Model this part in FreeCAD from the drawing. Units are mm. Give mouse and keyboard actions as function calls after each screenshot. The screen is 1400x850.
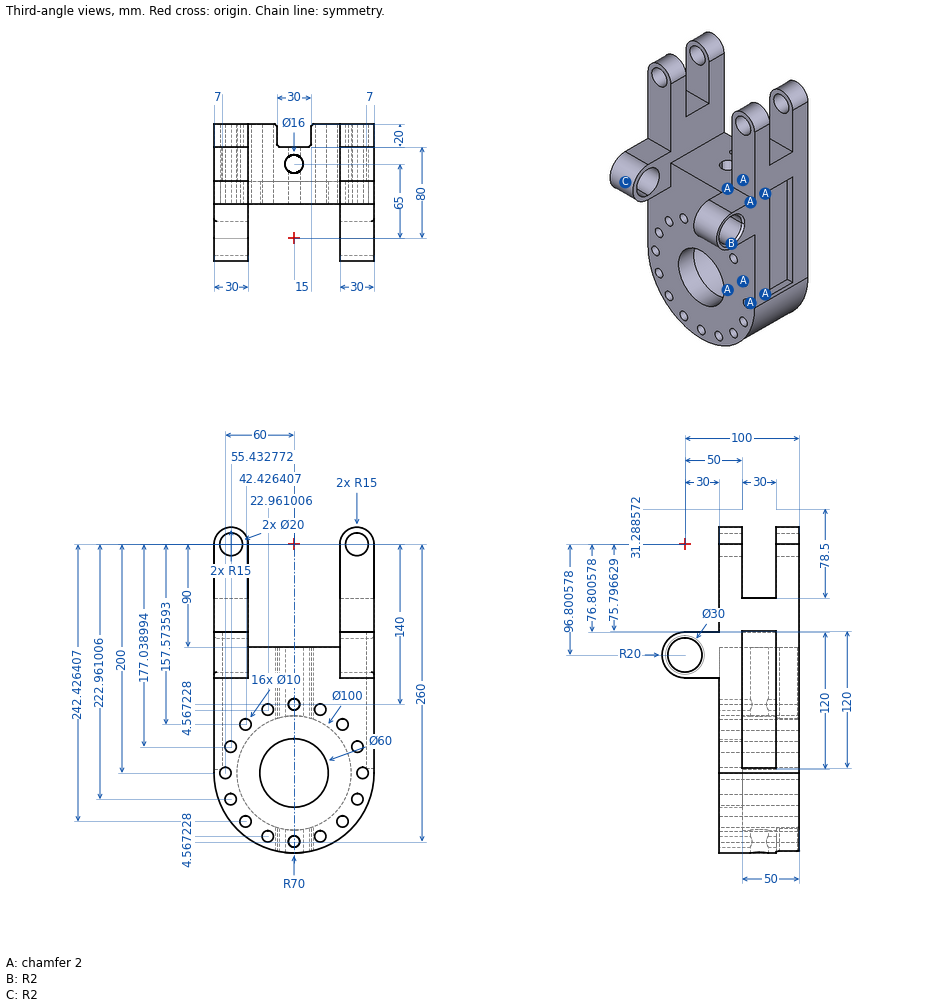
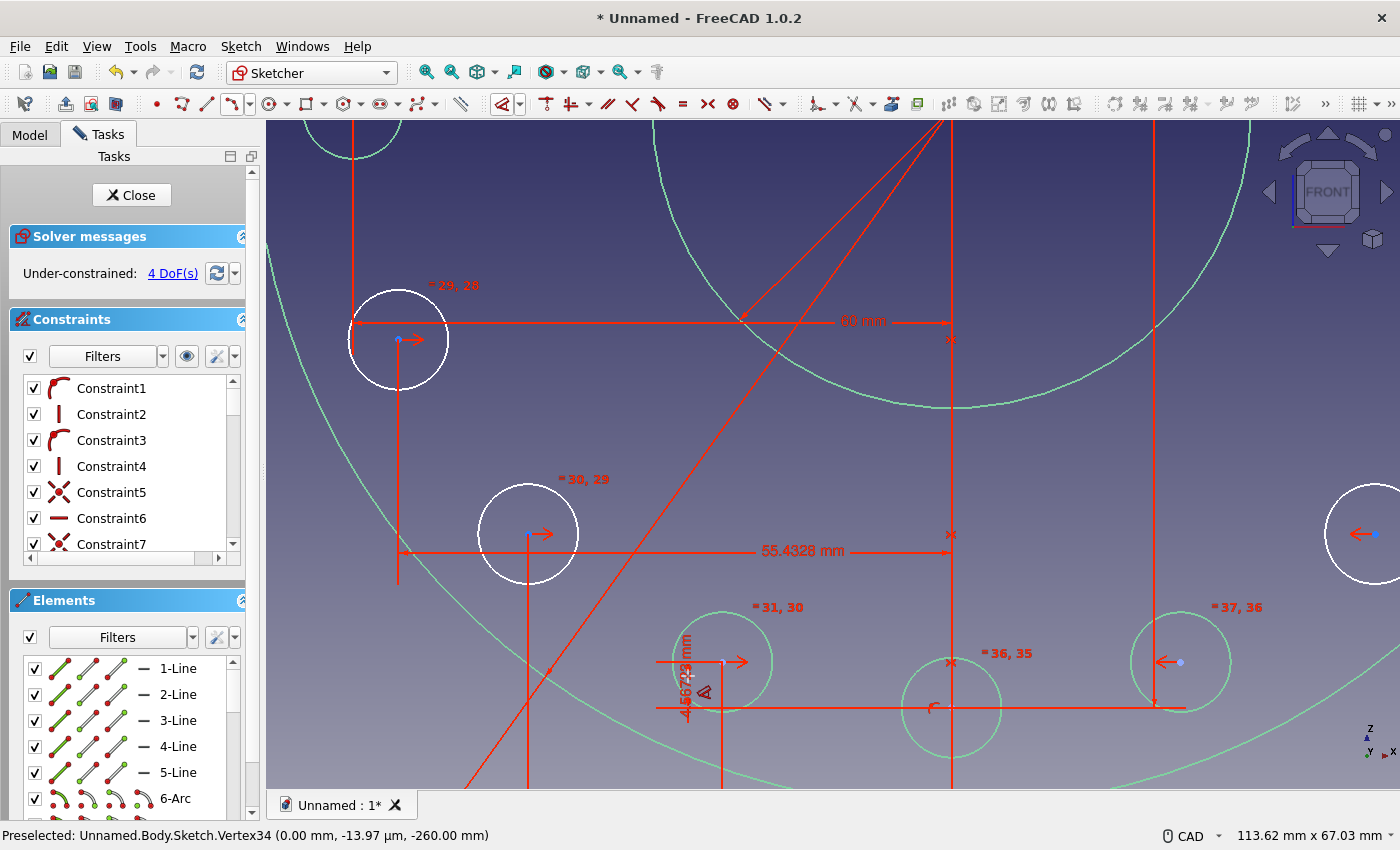
scroll(727, 666, down, 9)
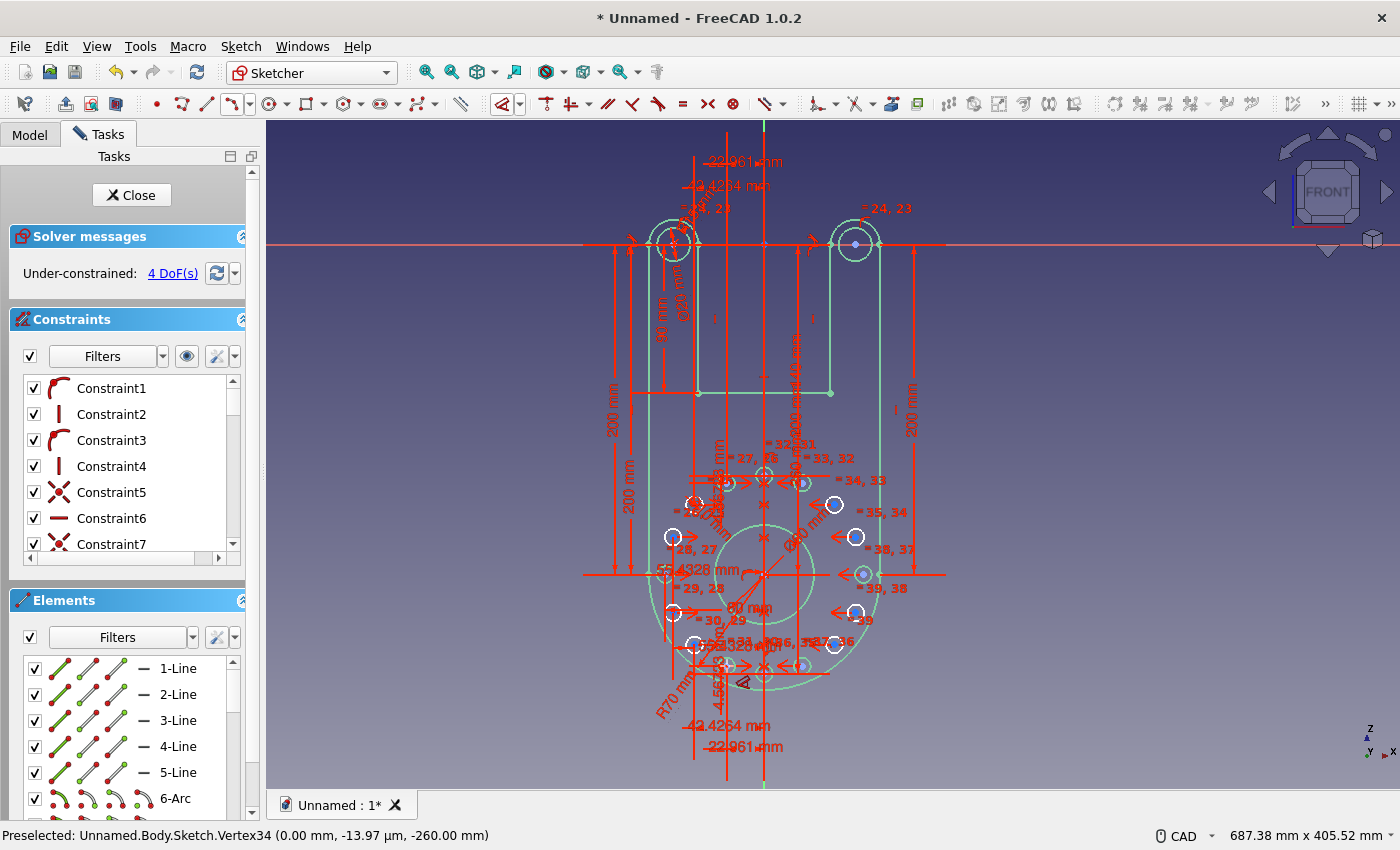
click(694, 505)
click(798, 315)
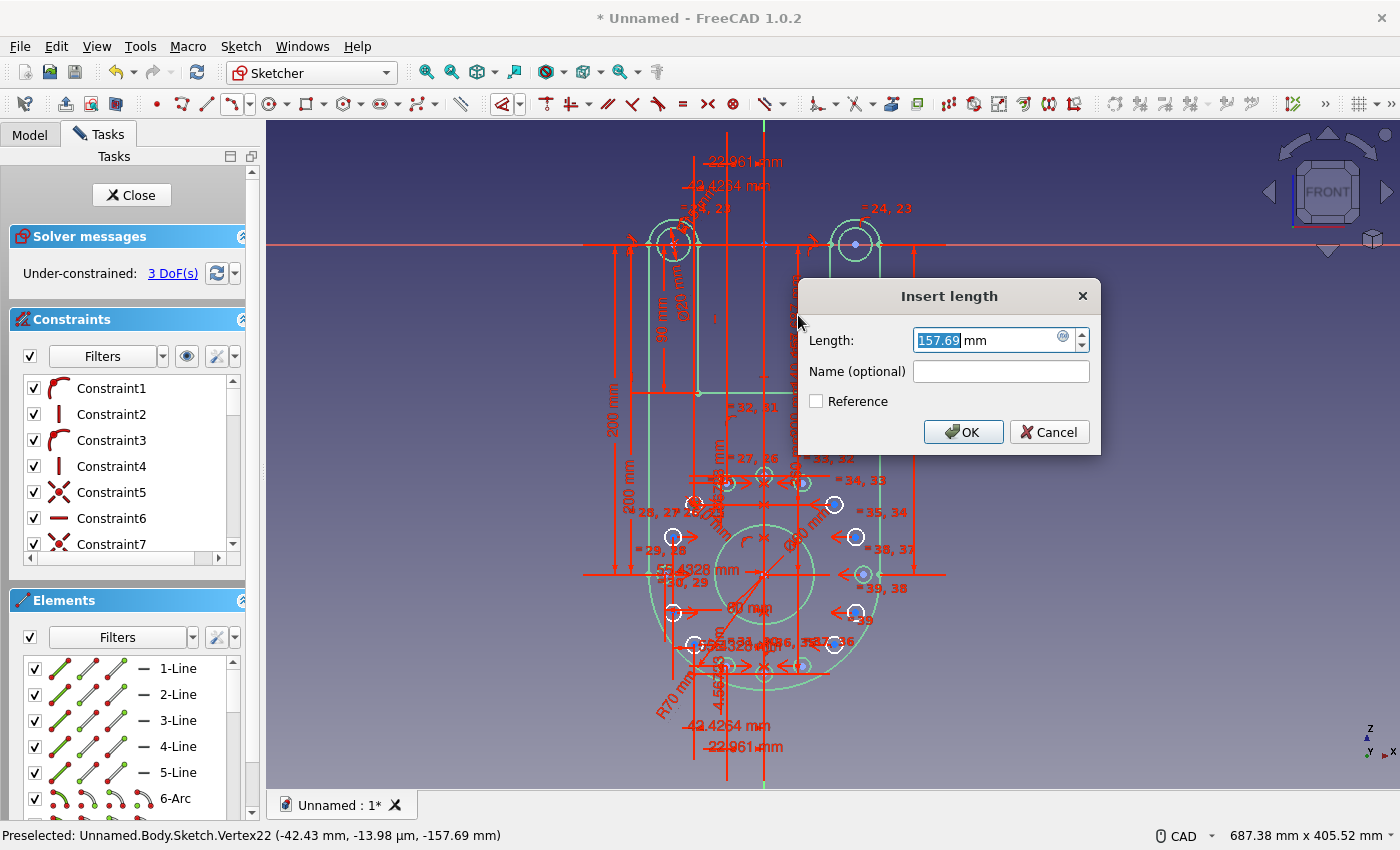
text(157.573593)
key(Return)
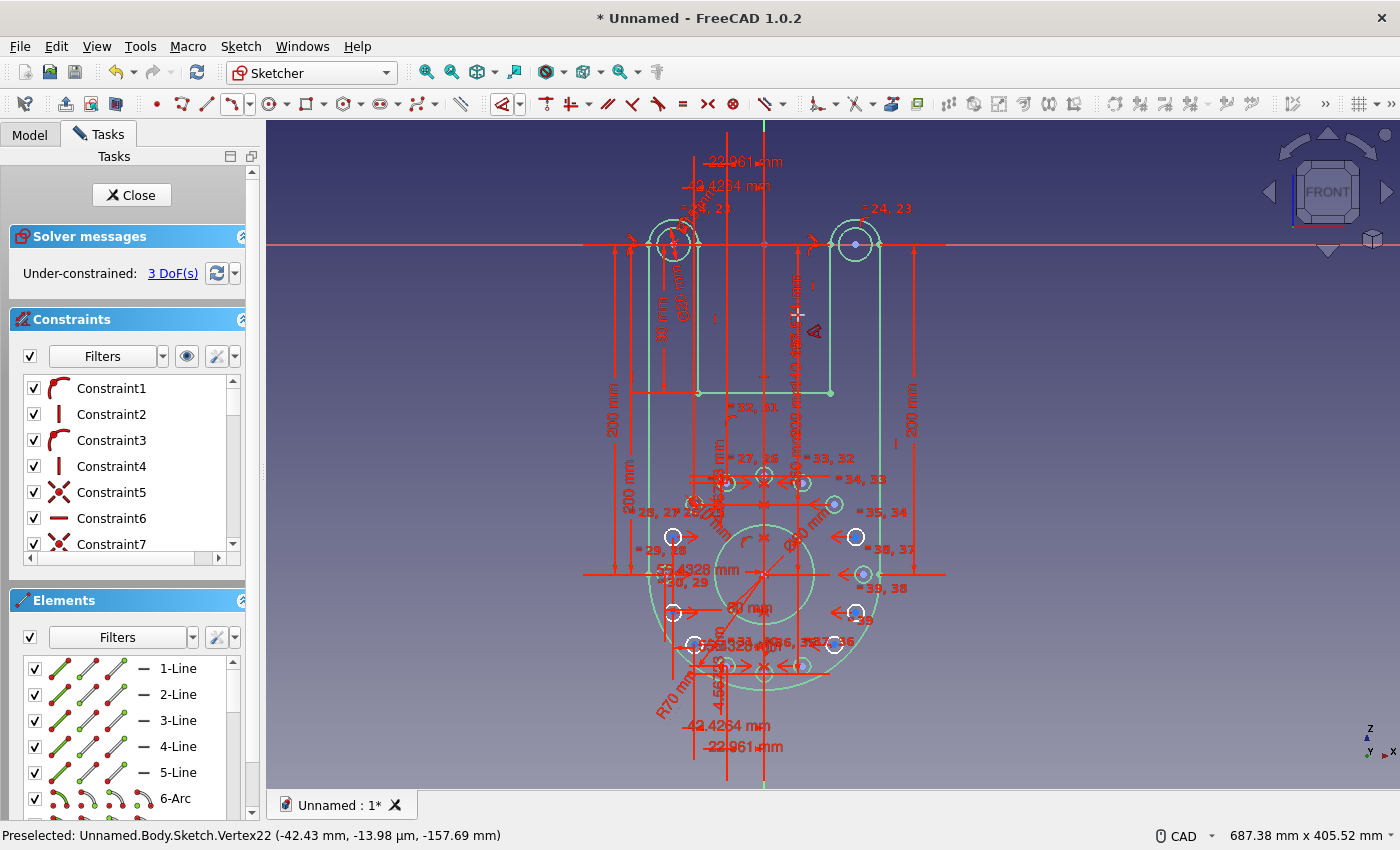
click(673, 537)
click(798, 289)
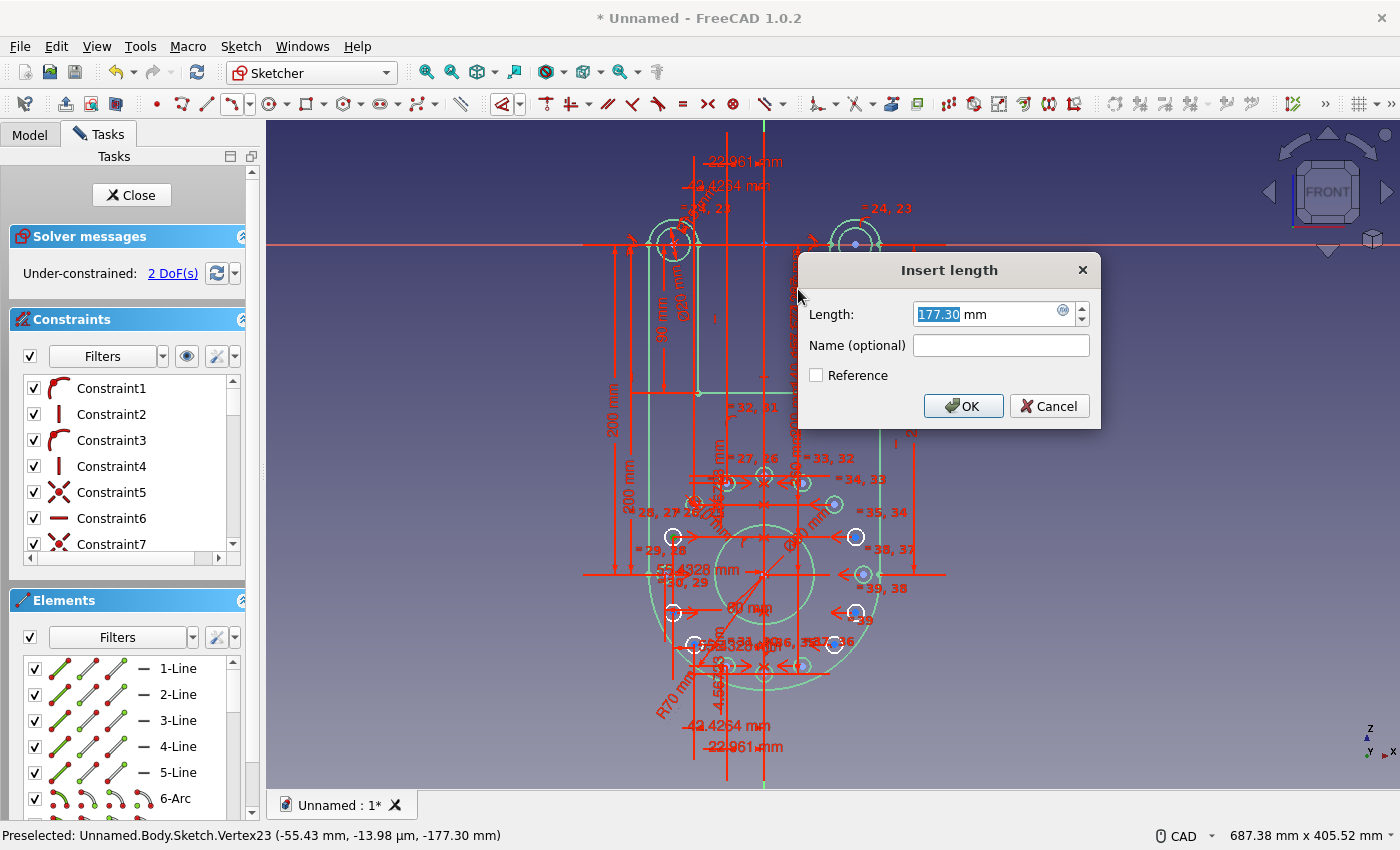
text(177.038994)
key(Return)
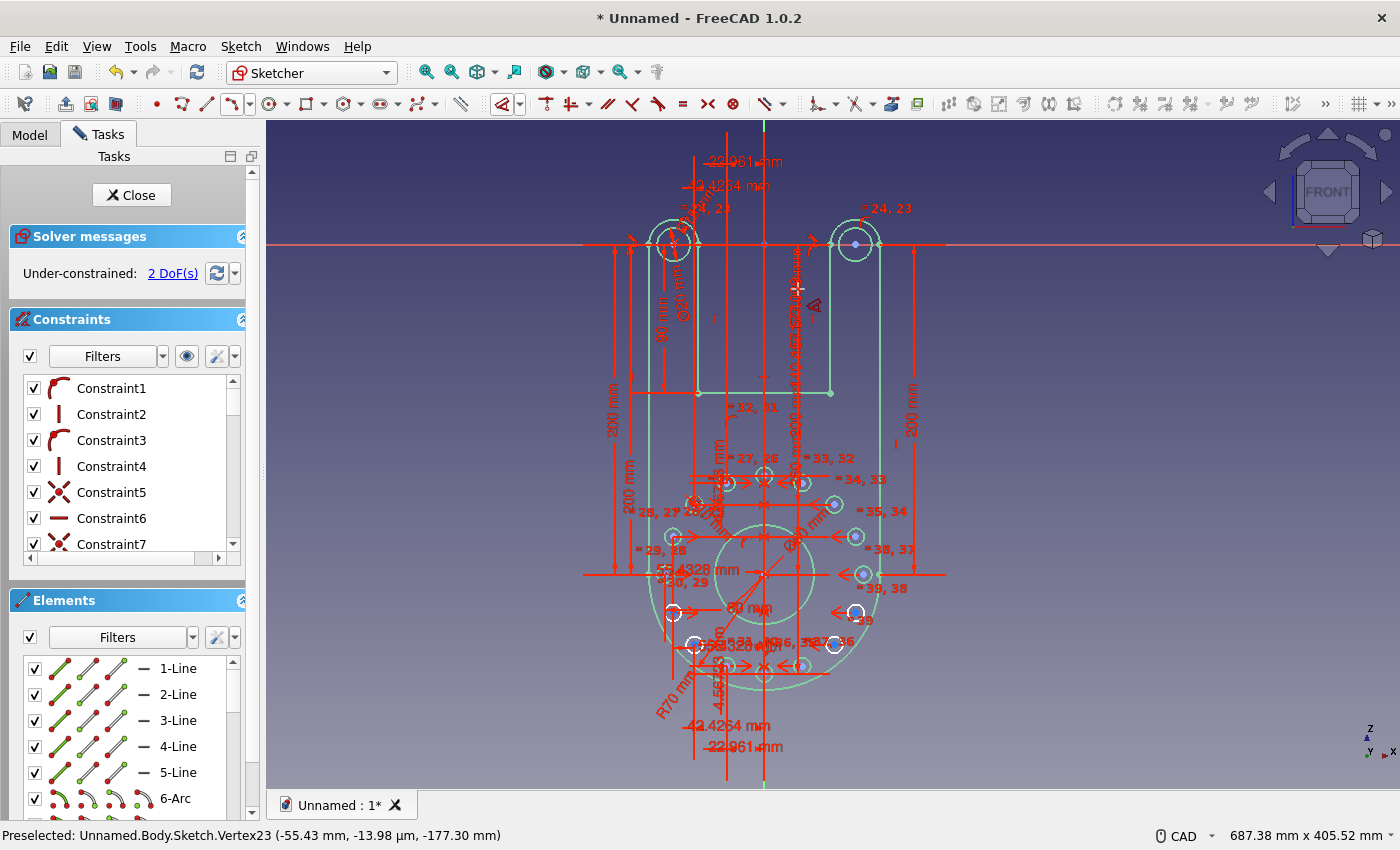
click(673, 613)
click(615, 344)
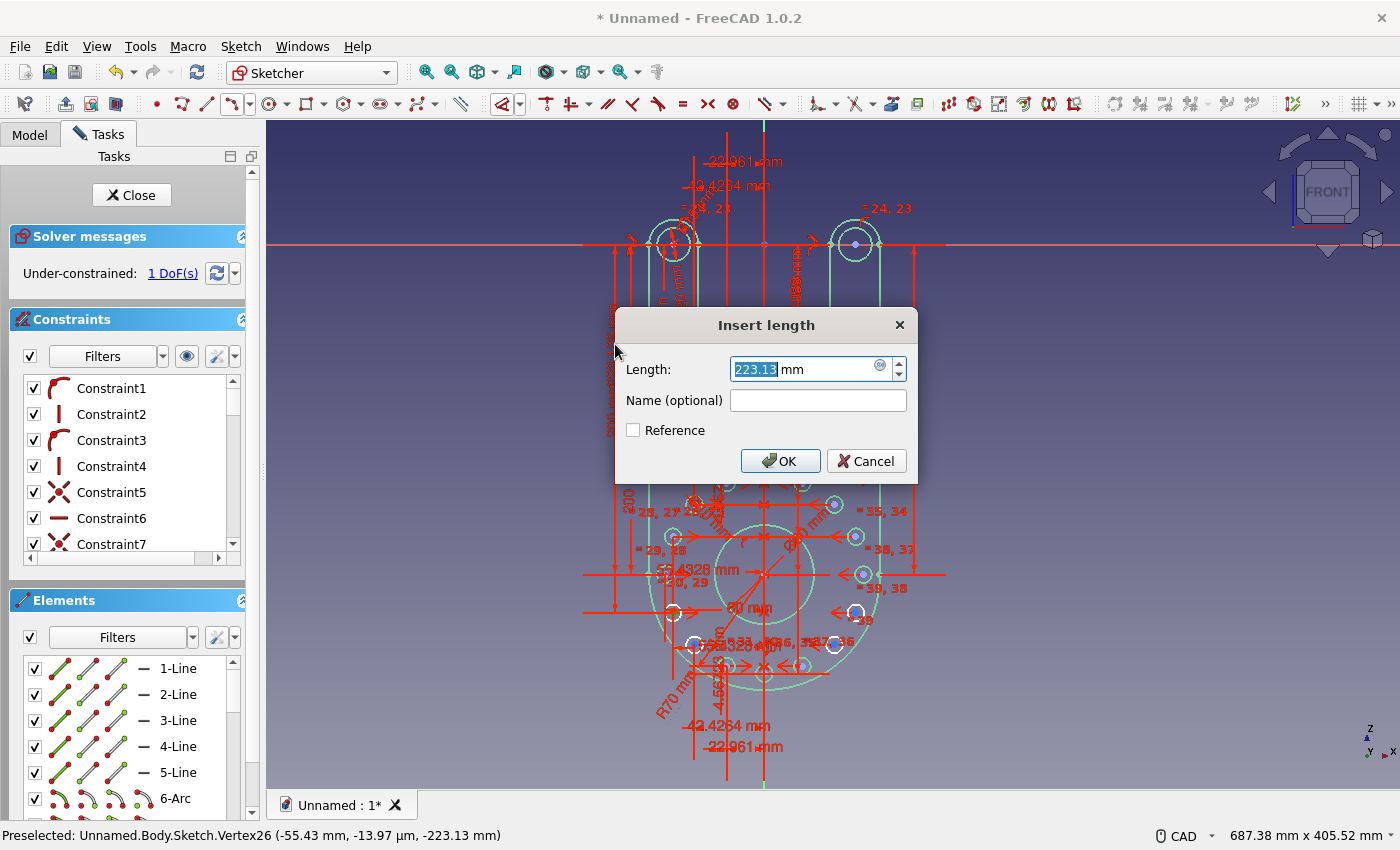
text(222.961006)
key(Return)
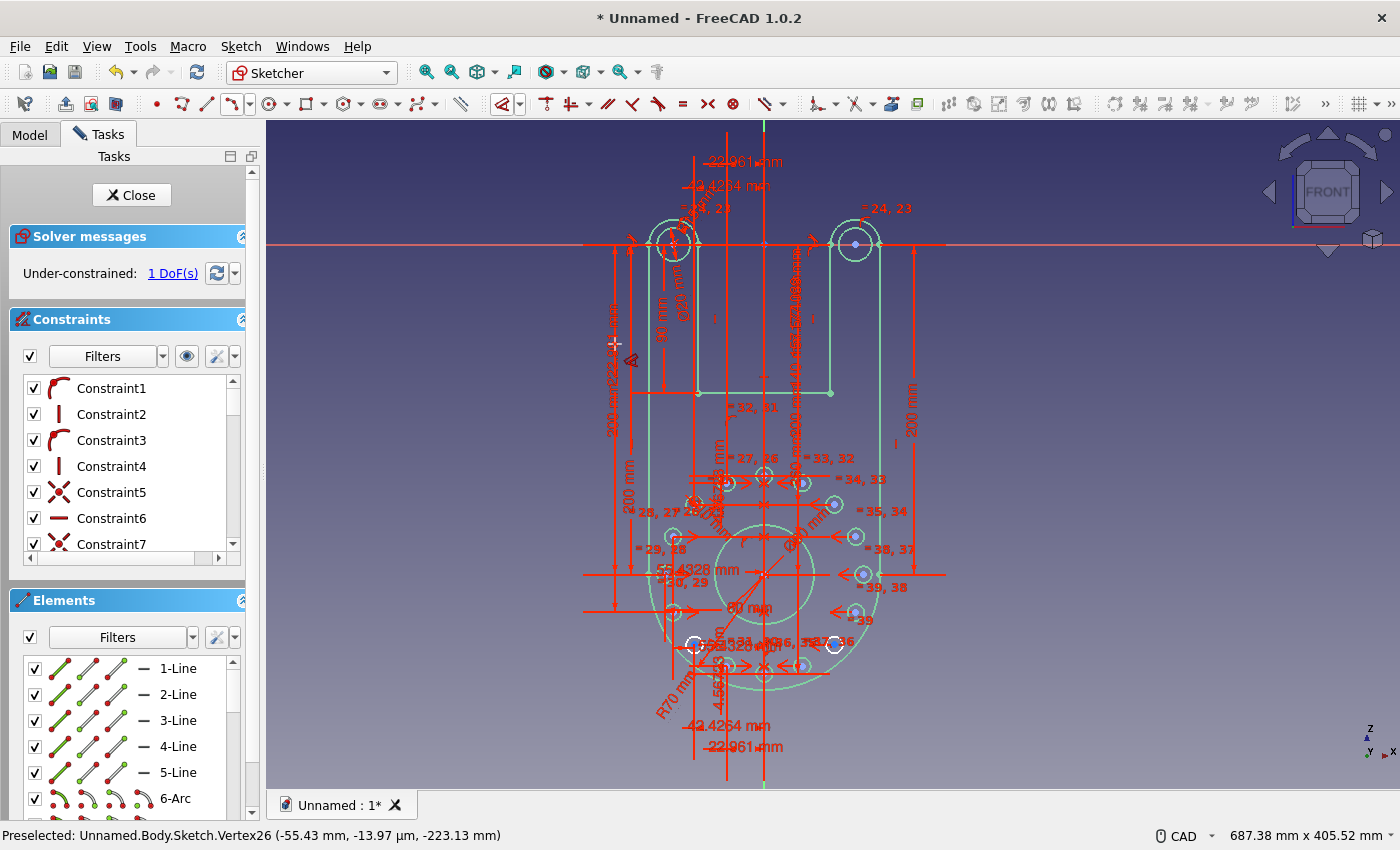
click(694, 645)
click(798, 585)